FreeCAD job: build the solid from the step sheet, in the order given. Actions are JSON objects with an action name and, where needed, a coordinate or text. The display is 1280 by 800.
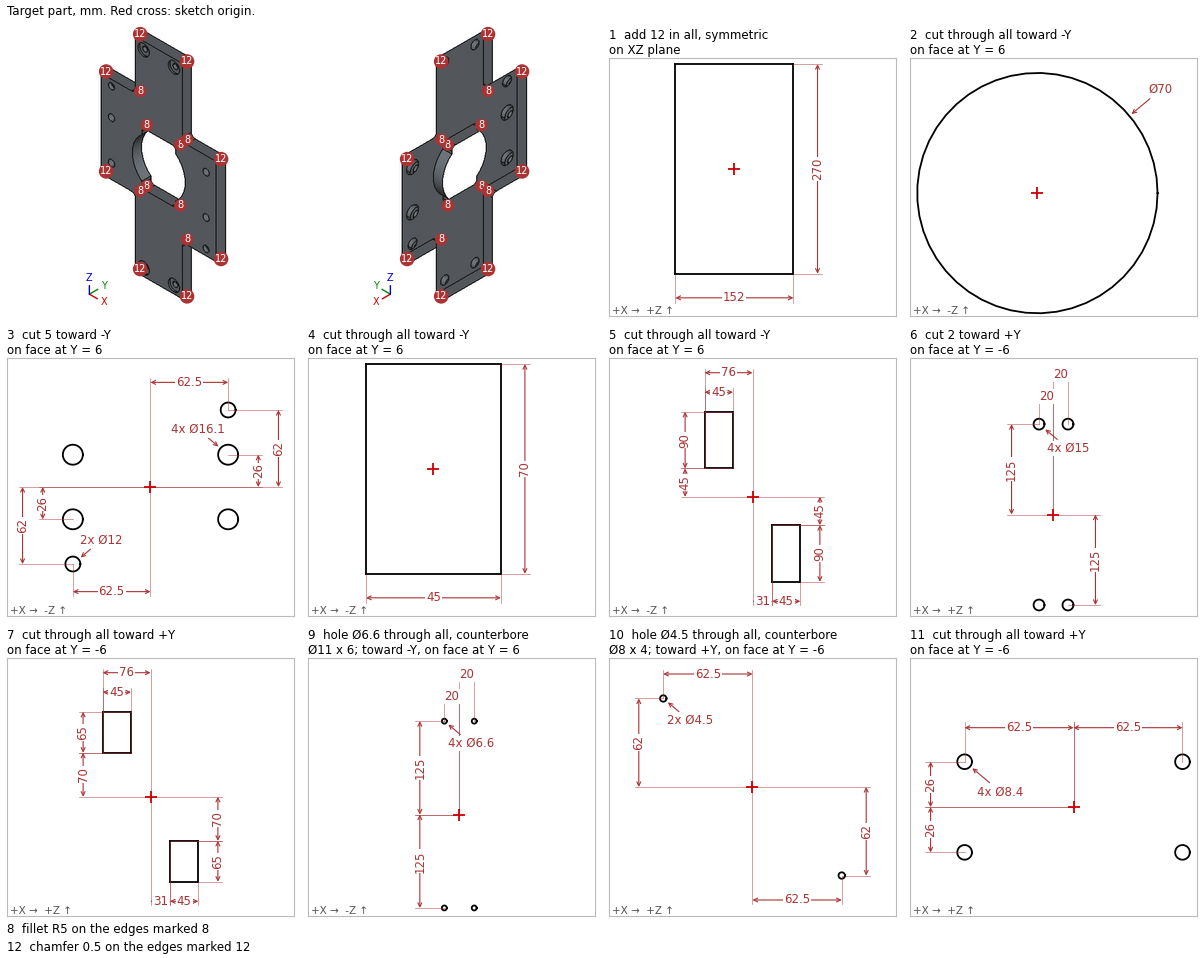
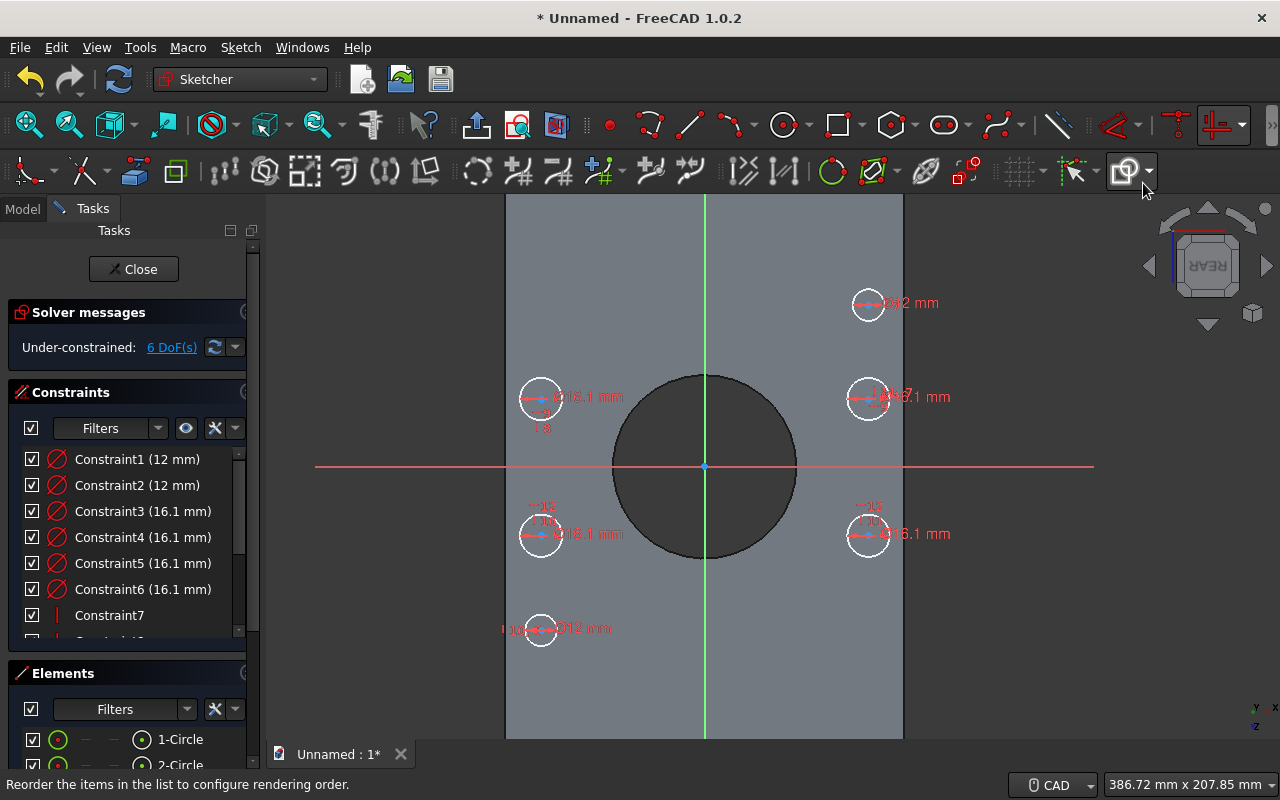
{"action": "key", "text": "d"}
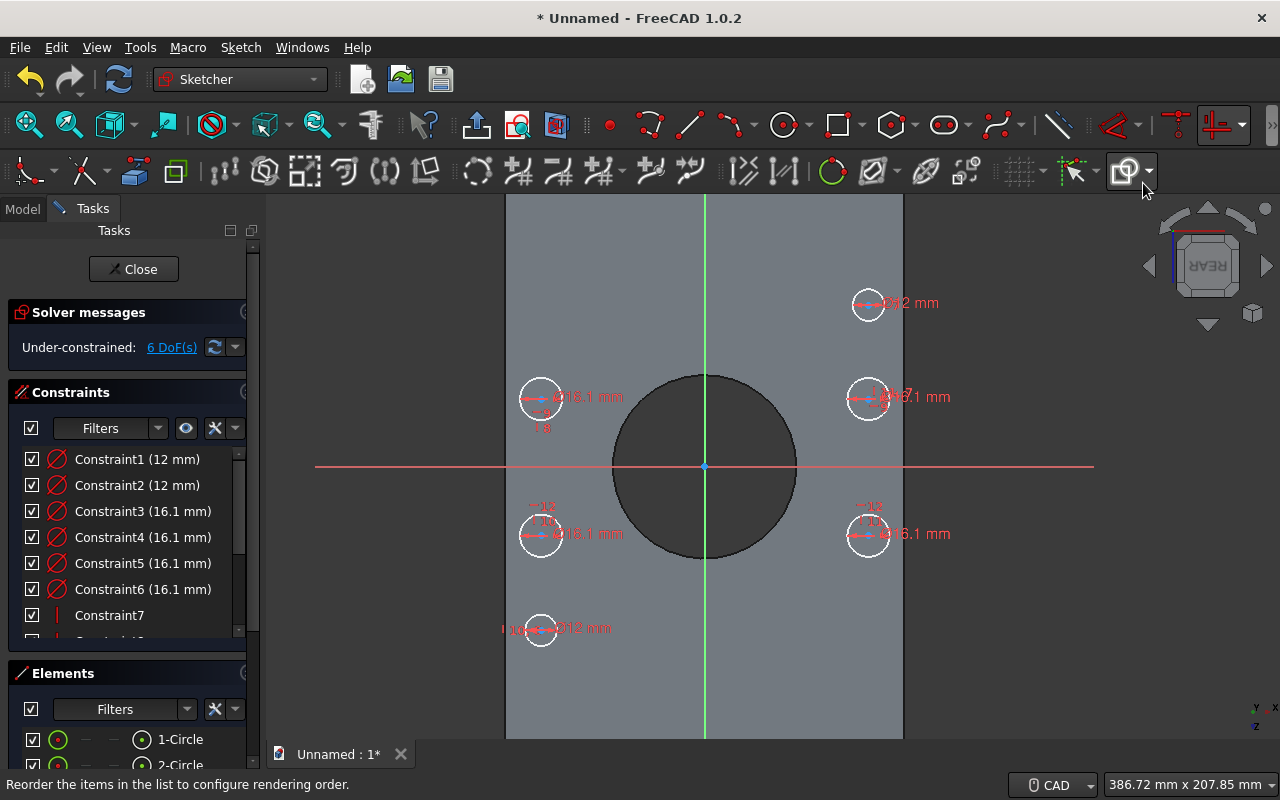
{"action": "left_click", "coordinate": [869, 305]}
{"action": "left_click", "coordinate": [903, 386]}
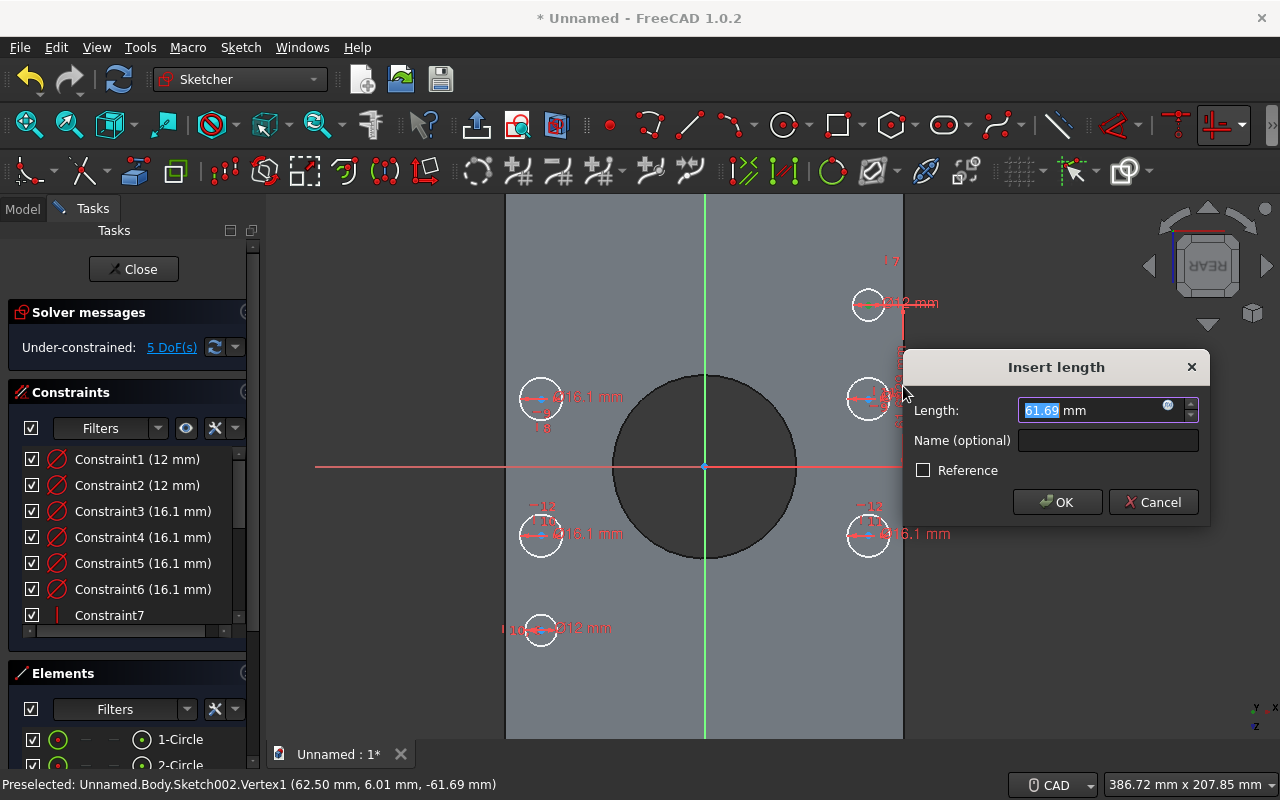
{"action": "type", "text": "62"}
{"action": "key", "text": "Return"}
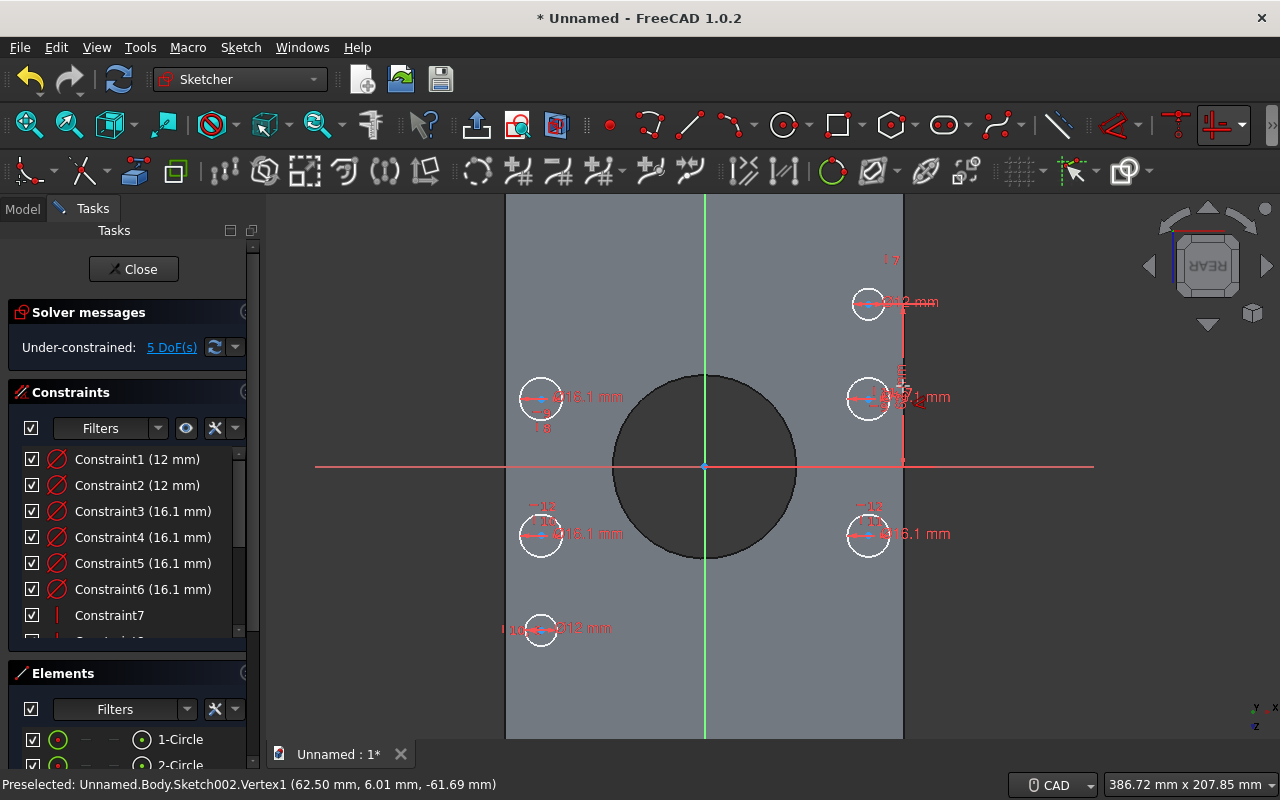
{"action": "left_click", "coordinate": [541, 630]}
{"action": "left_click", "coordinate": [507, 549]}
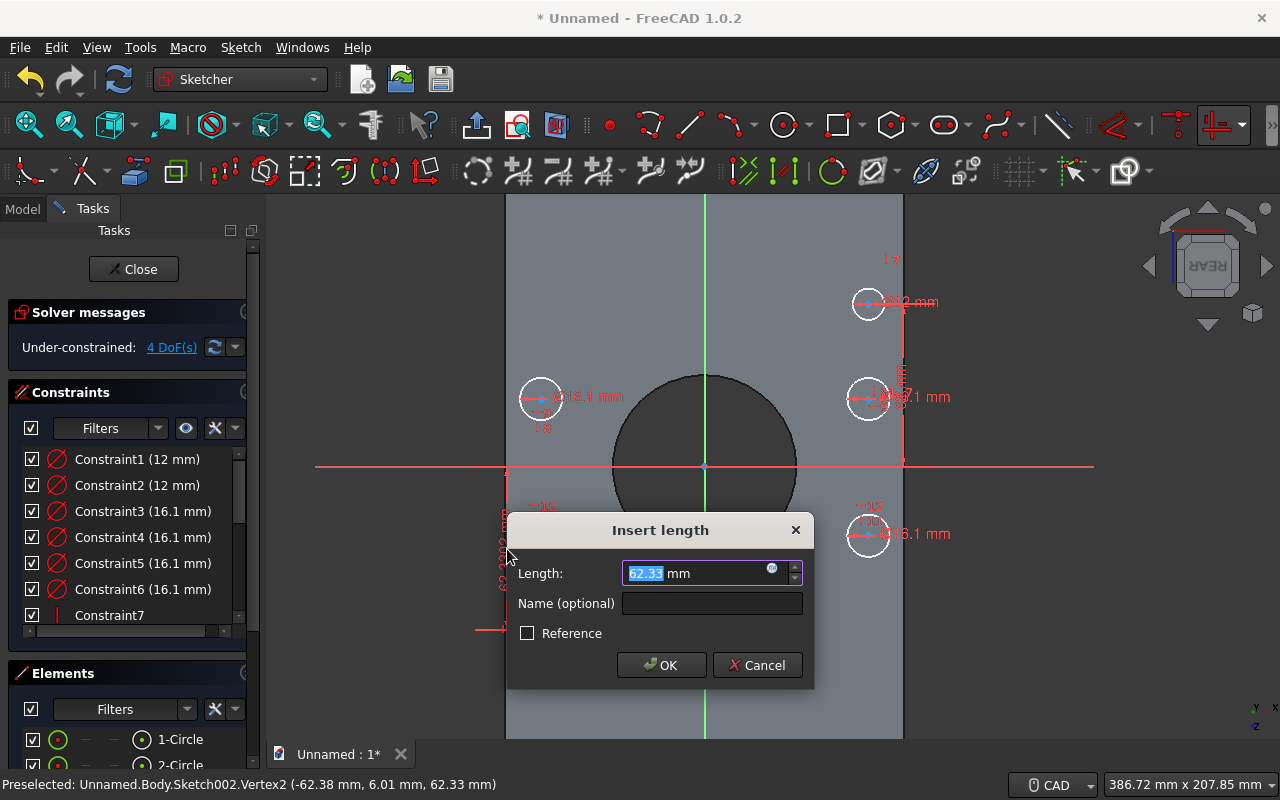
{"action": "type", "text": "62"}
{"action": "key", "text": "Return"}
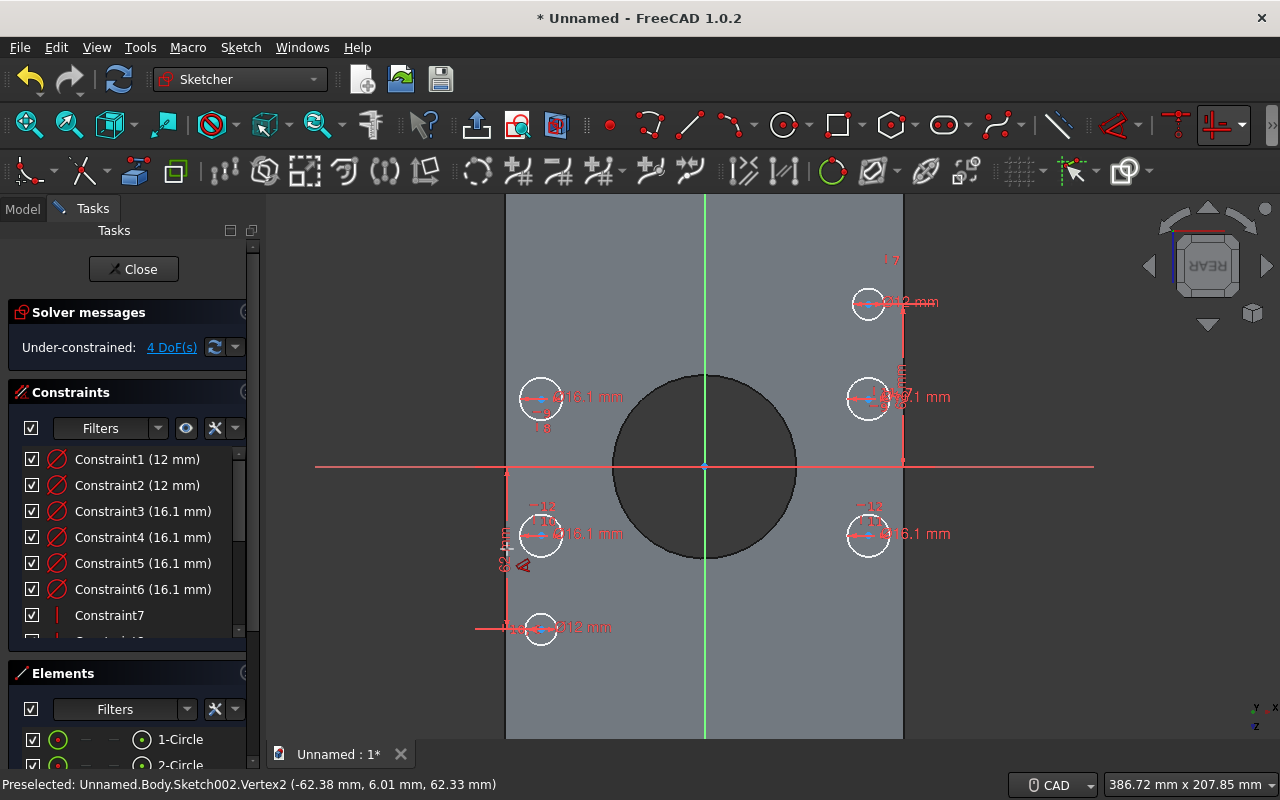
{"action": "left_click", "coordinate": [869, 399]}
{"action": "left_click", "coordinate": [903, 433]}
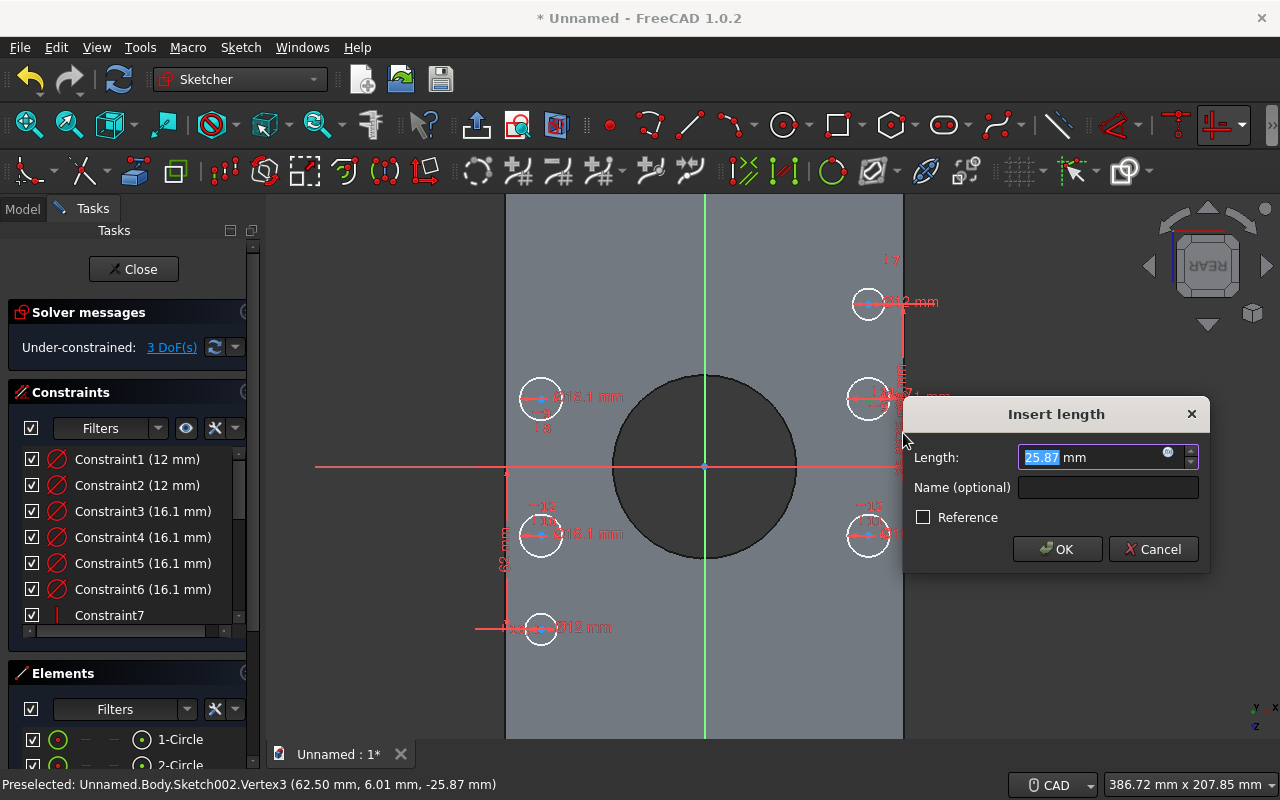
{"action": "type", "text": "26"}
{"action": "key", "text": "Return"}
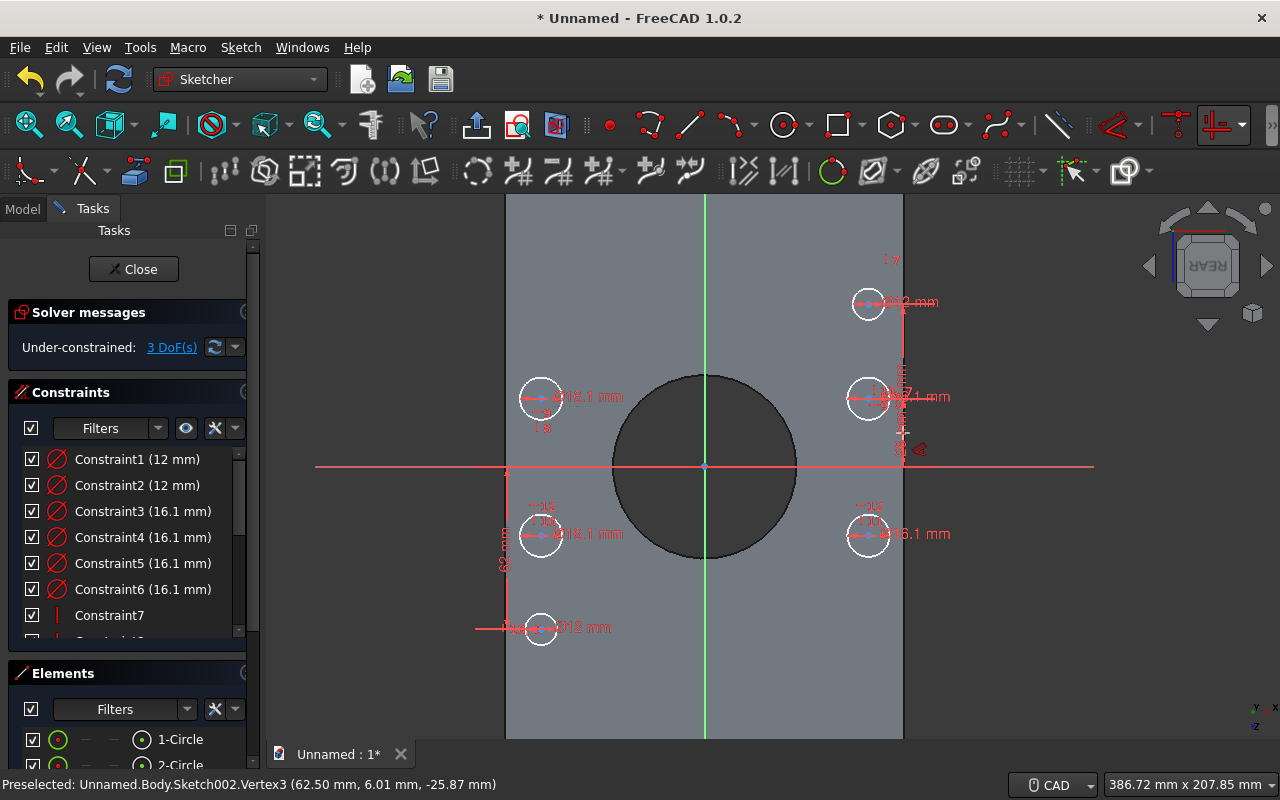
{"action": "left_click", "coordinate": [541, 536]}
{"action": "left_click", "coordinate": [507, 501]}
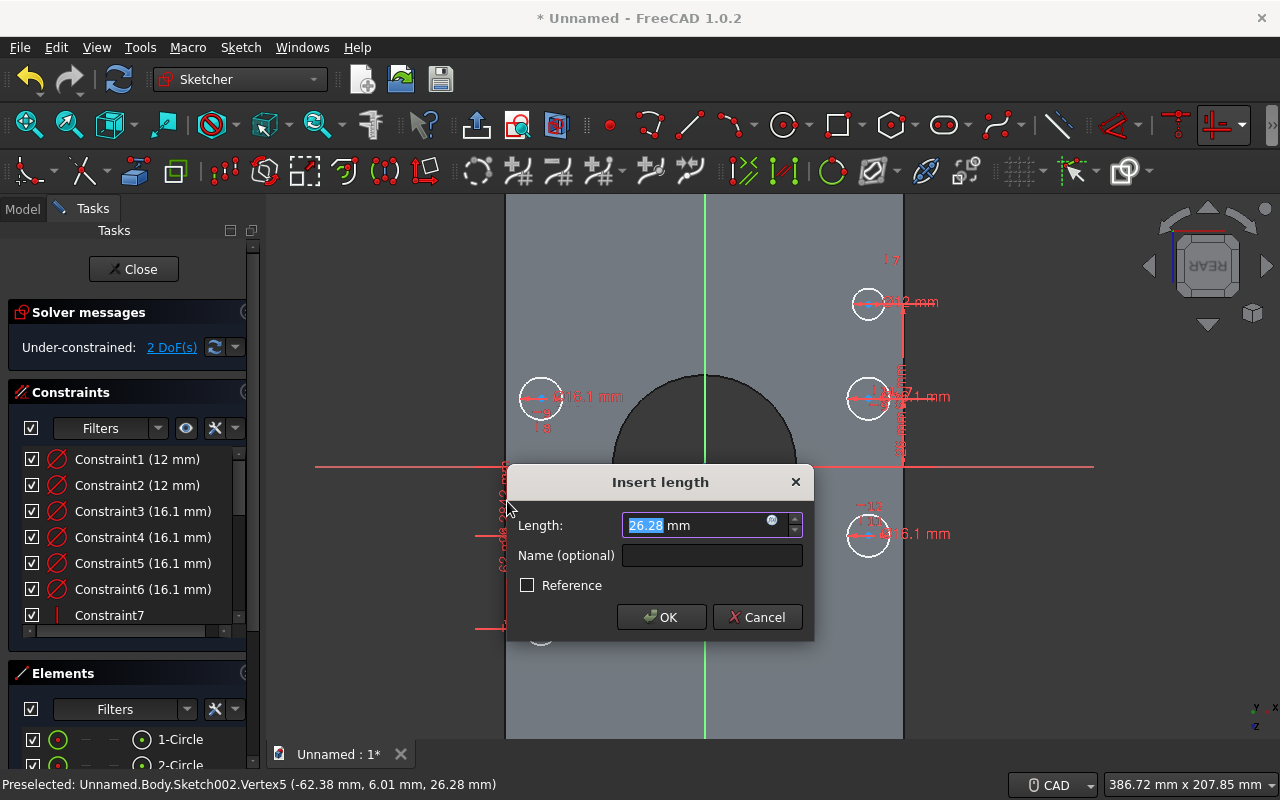
{"action": "type", "text": "26"}
{"action": "key", "text": "Return"}